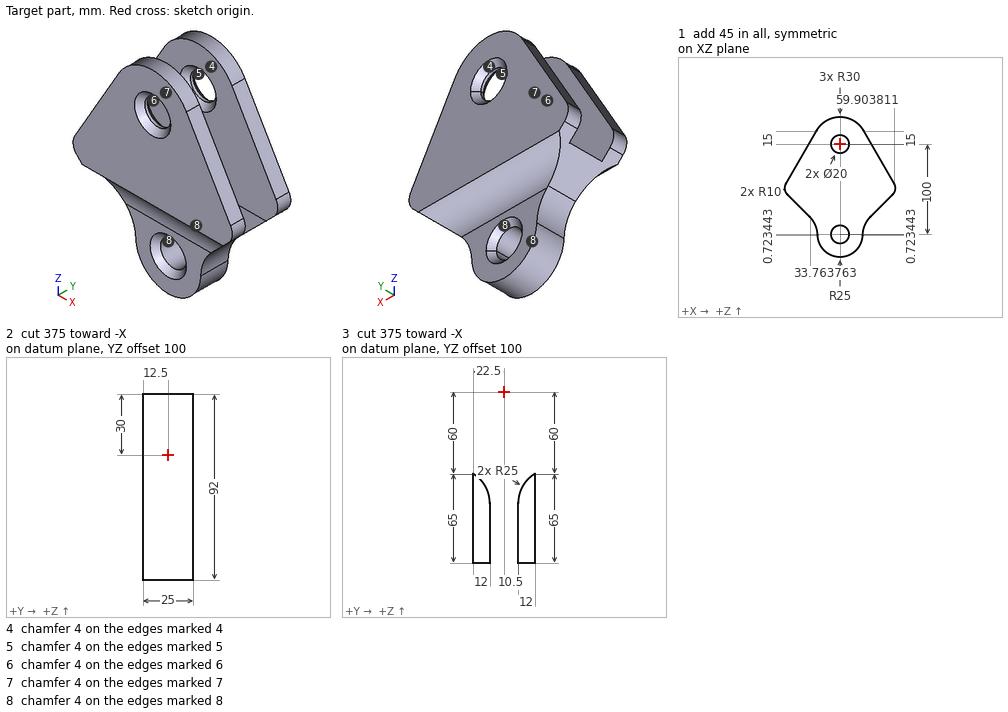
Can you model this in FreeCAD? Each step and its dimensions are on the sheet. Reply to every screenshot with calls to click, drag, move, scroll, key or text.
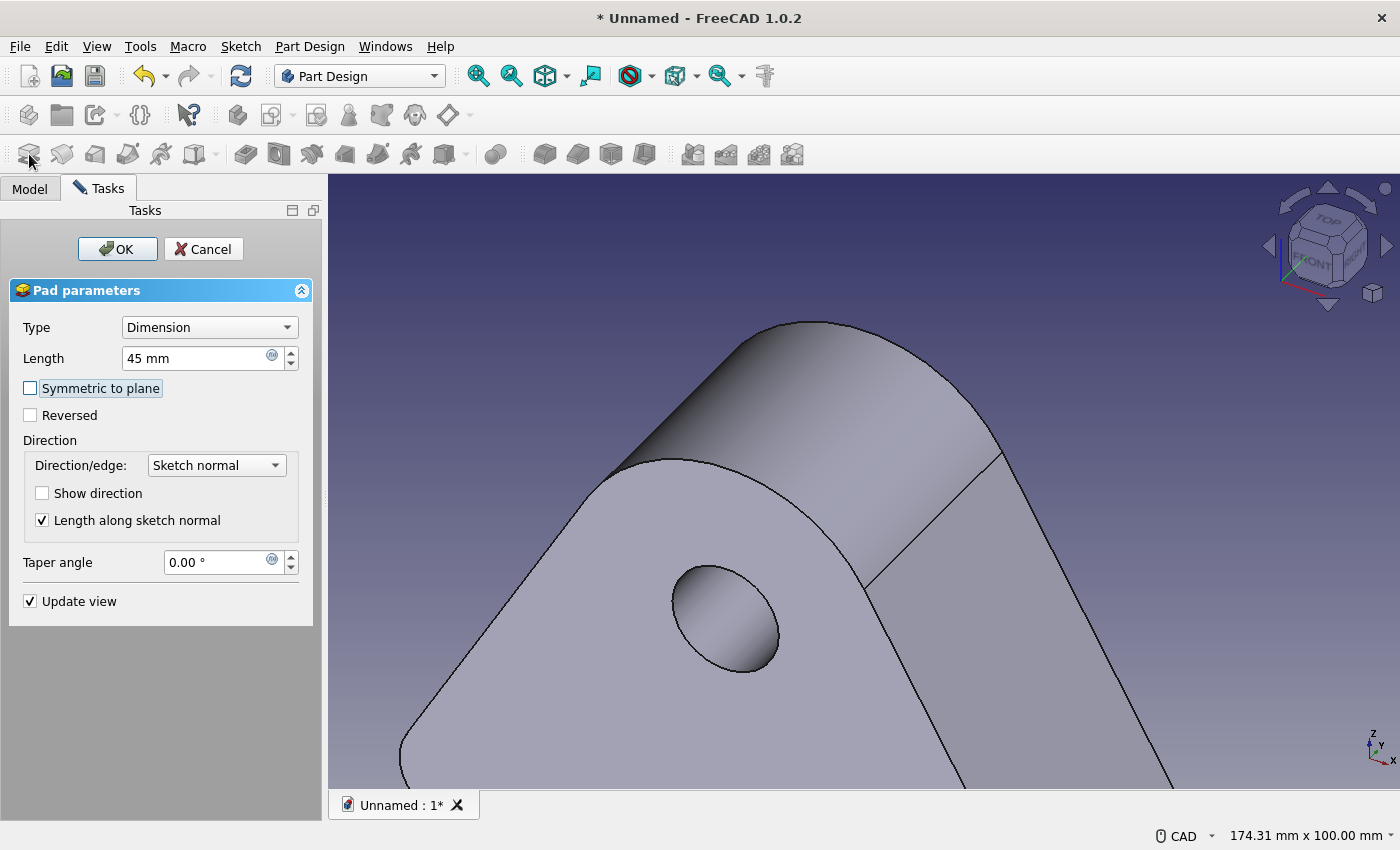
click(31, 388)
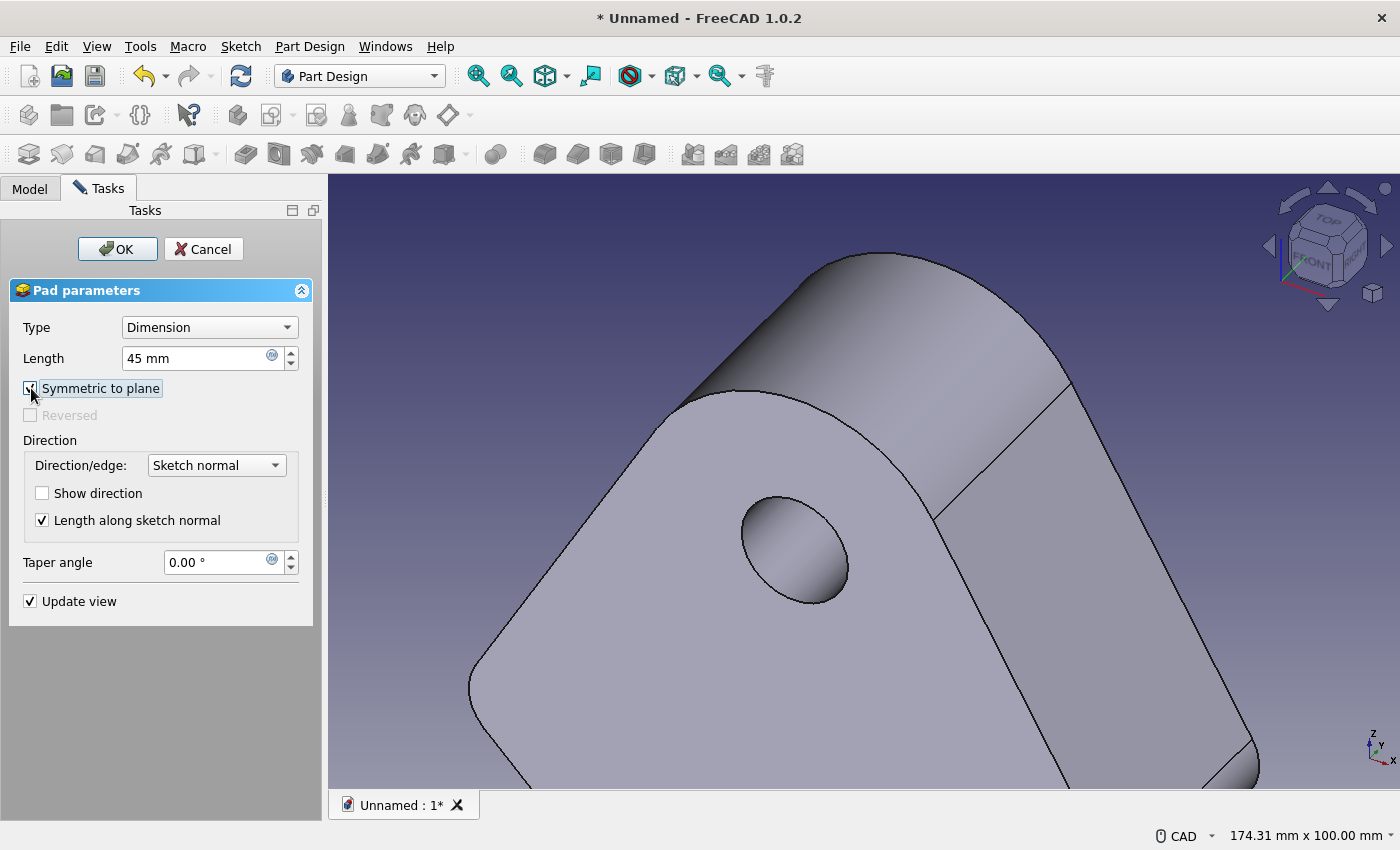
click(118, 249)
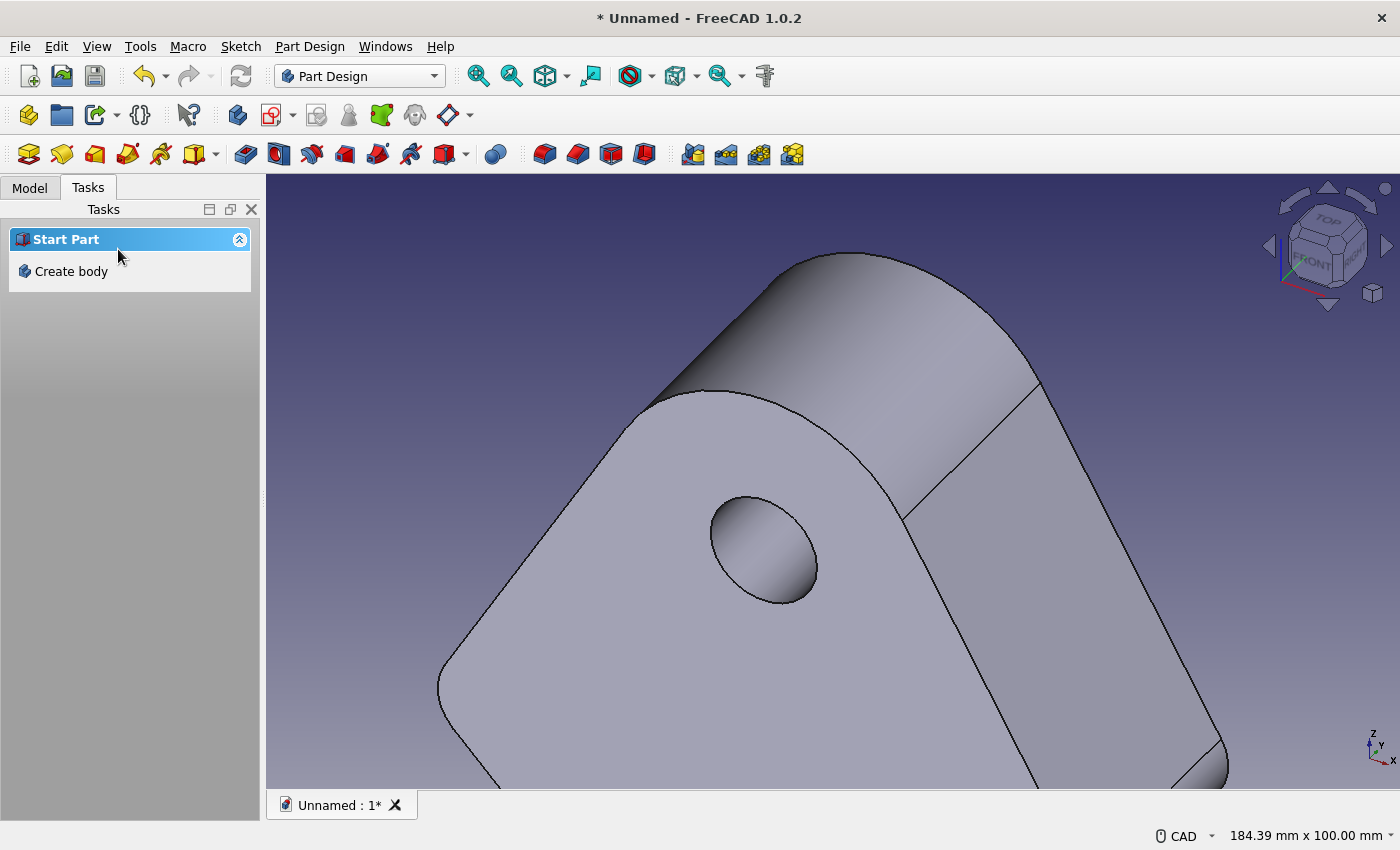
click(479, 76)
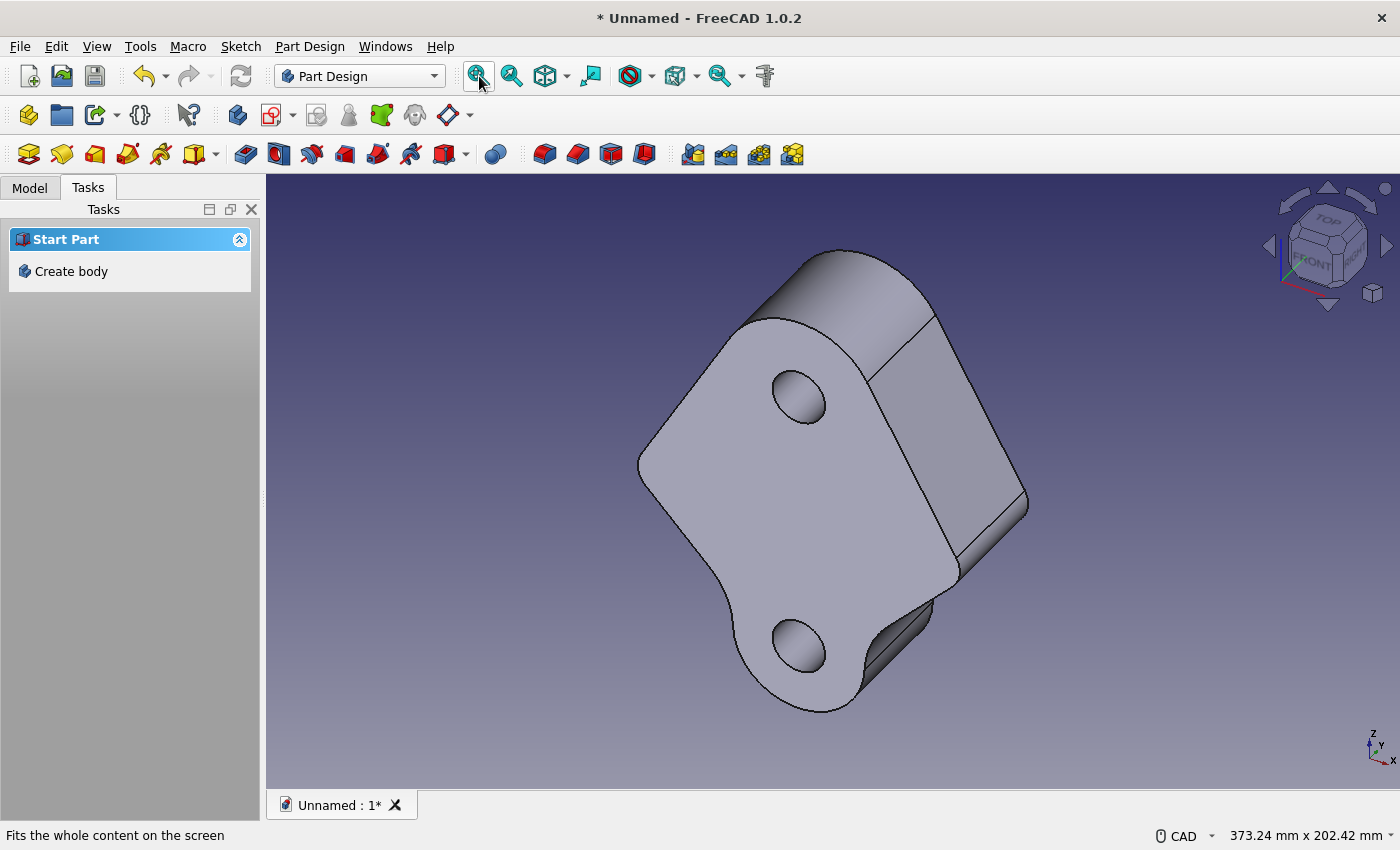
click(30, 188)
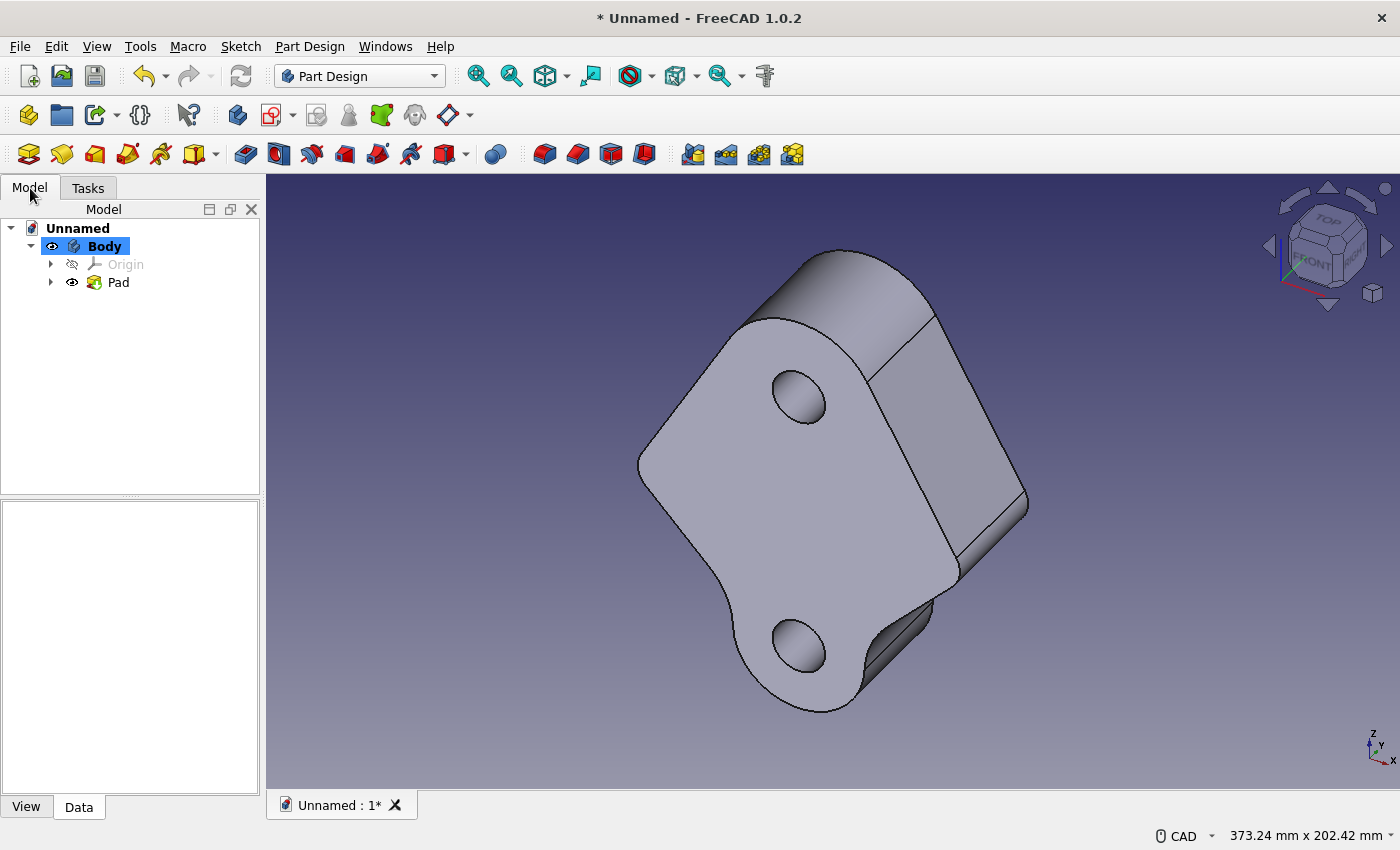
click(51, 264)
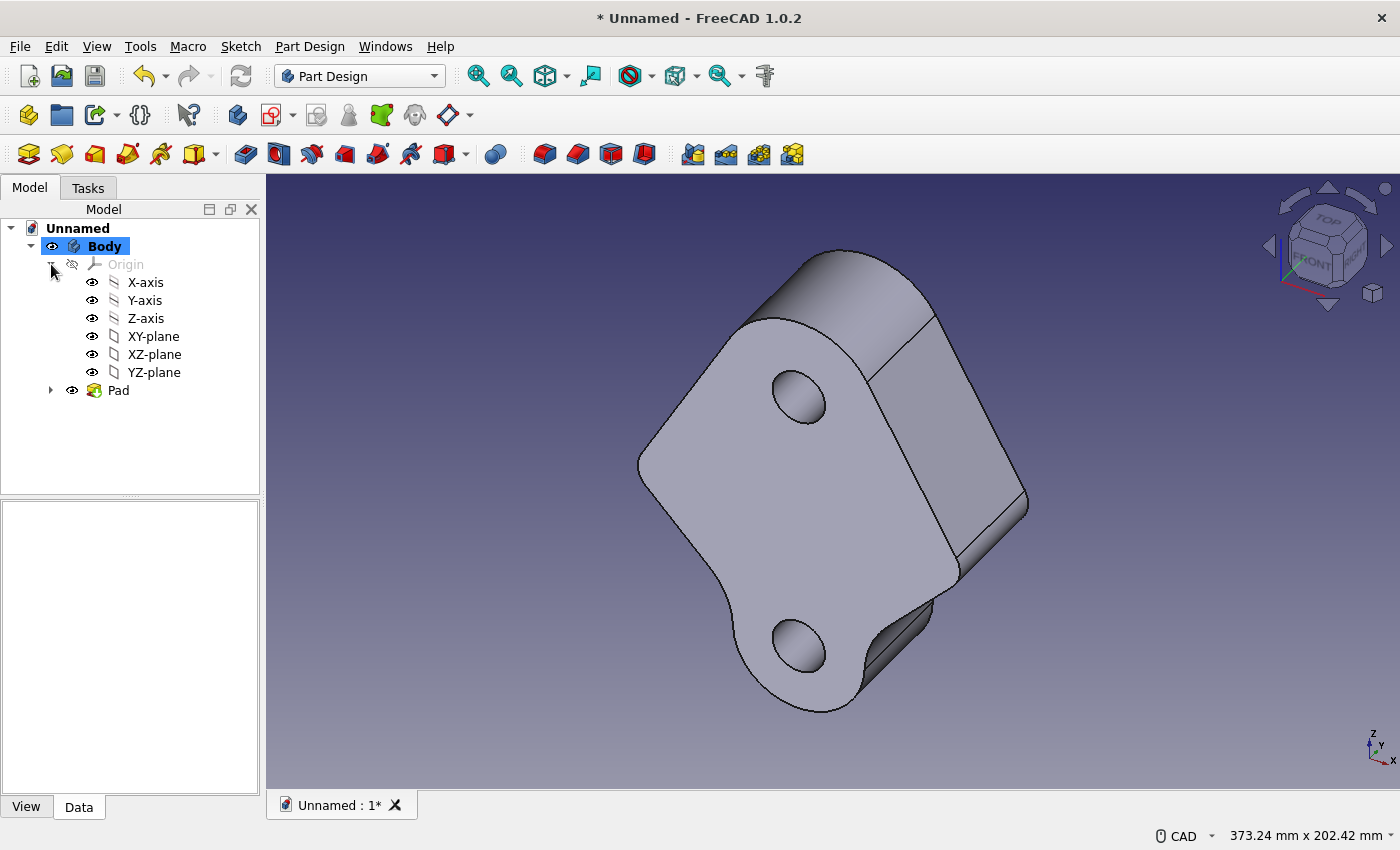
click(137, 372)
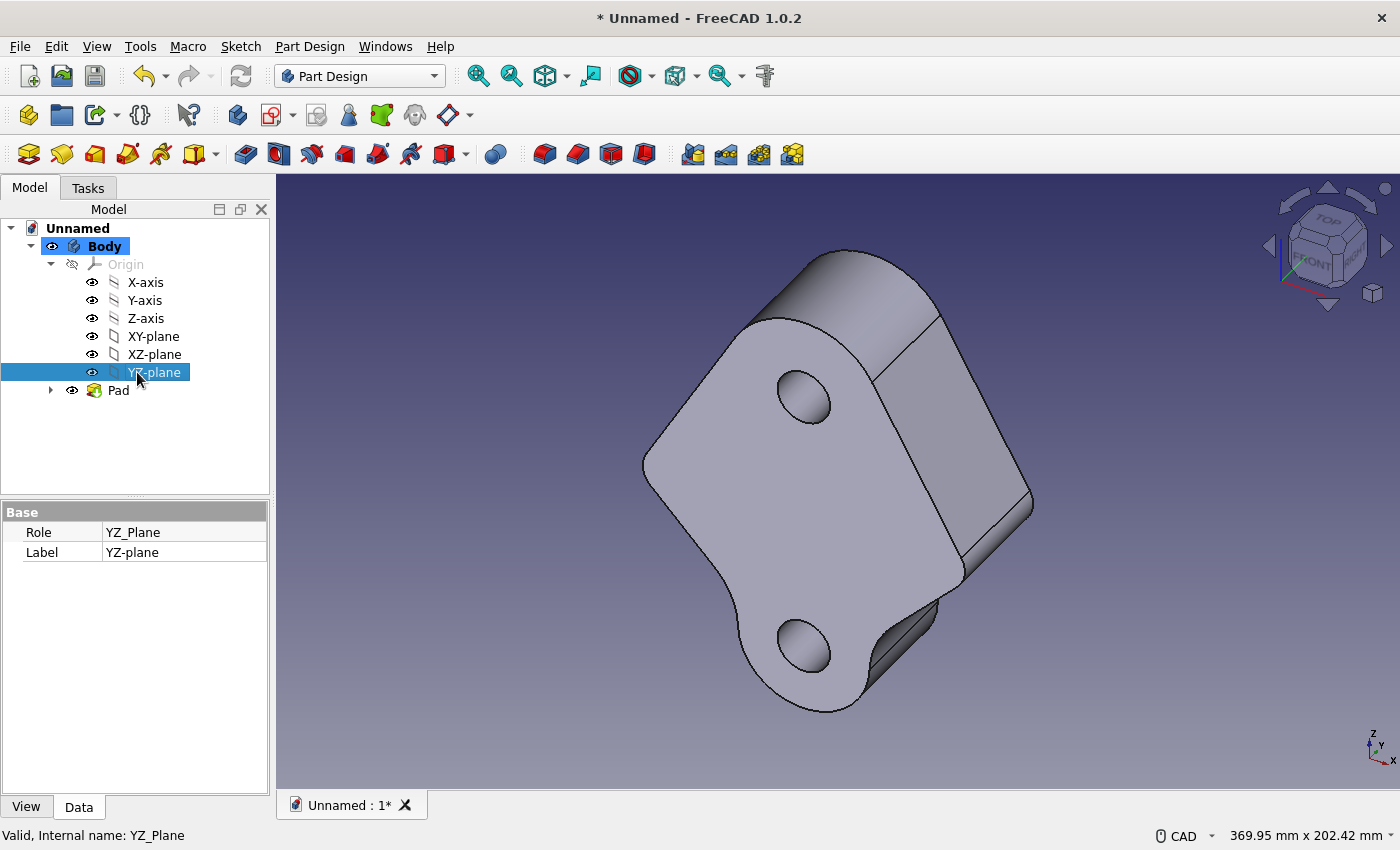
click(448, 116)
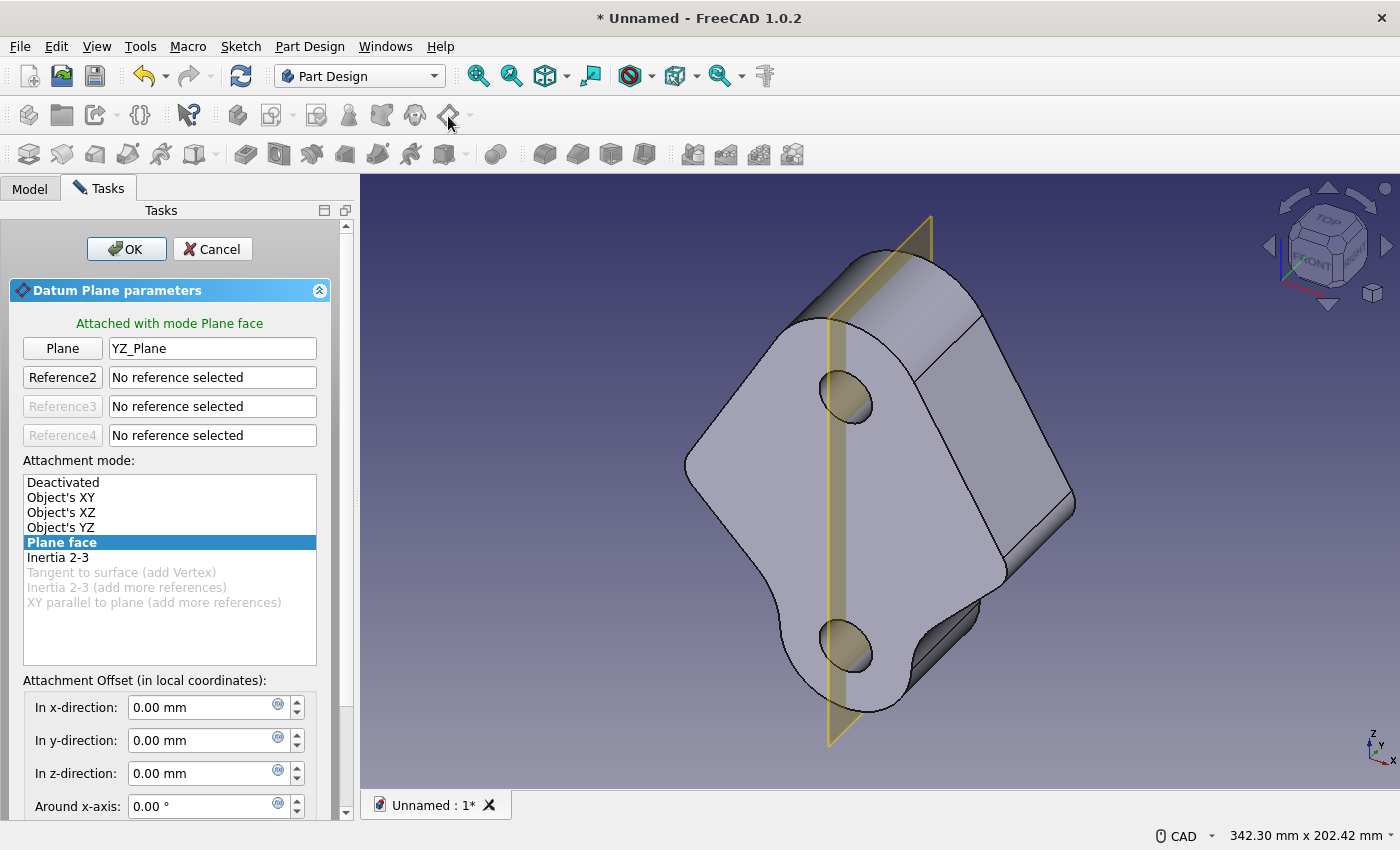
triple_click(210, 774)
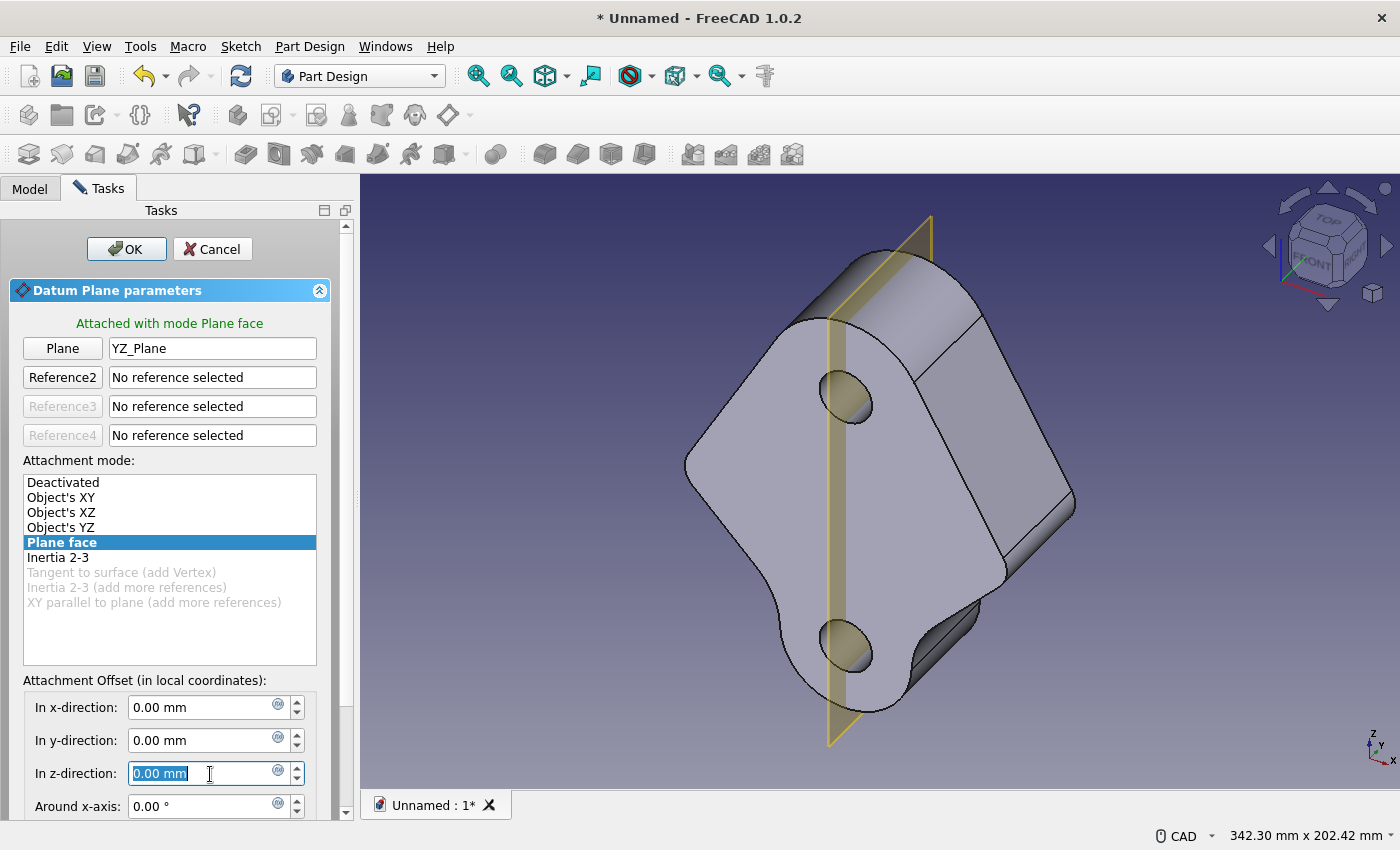
text(100)
key(Tab)